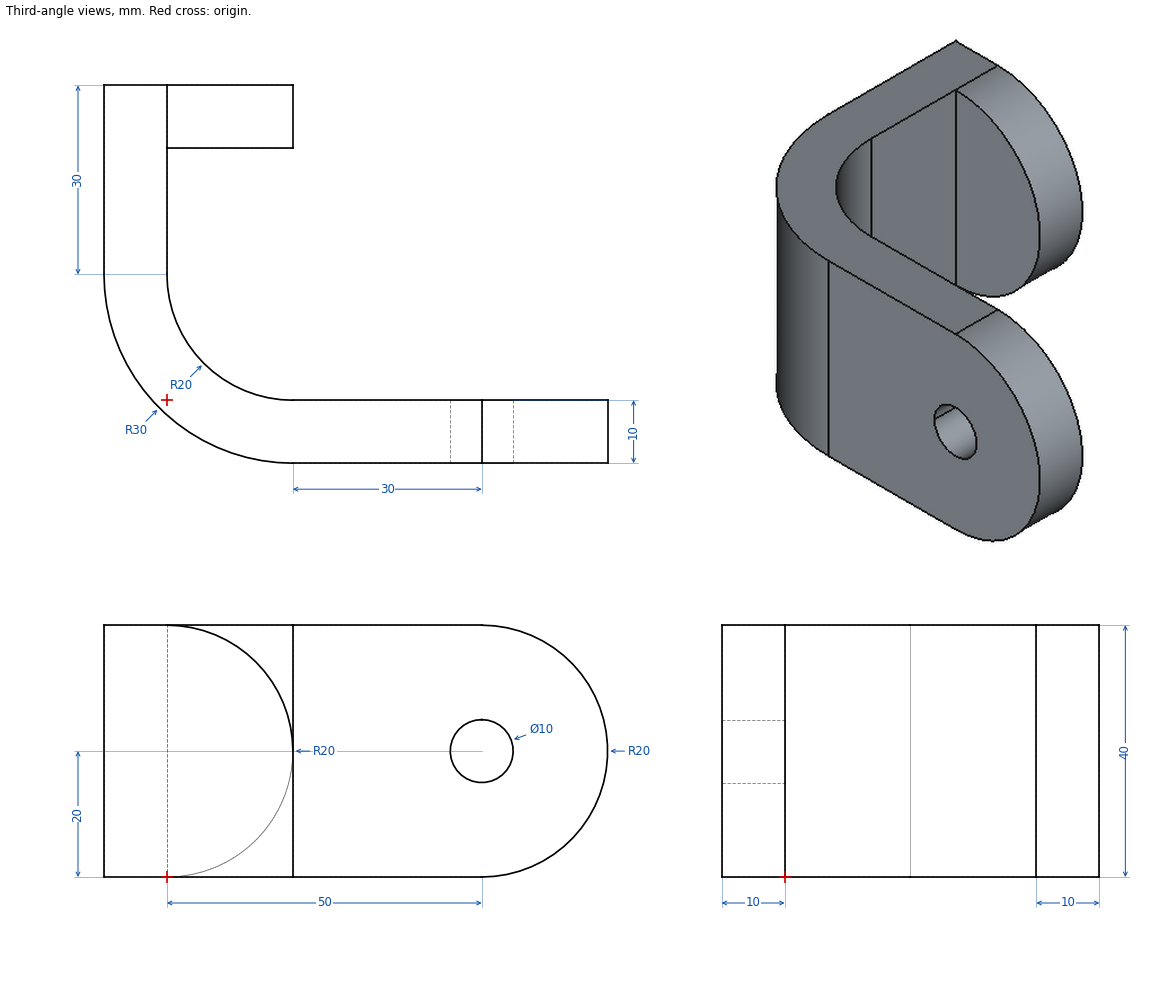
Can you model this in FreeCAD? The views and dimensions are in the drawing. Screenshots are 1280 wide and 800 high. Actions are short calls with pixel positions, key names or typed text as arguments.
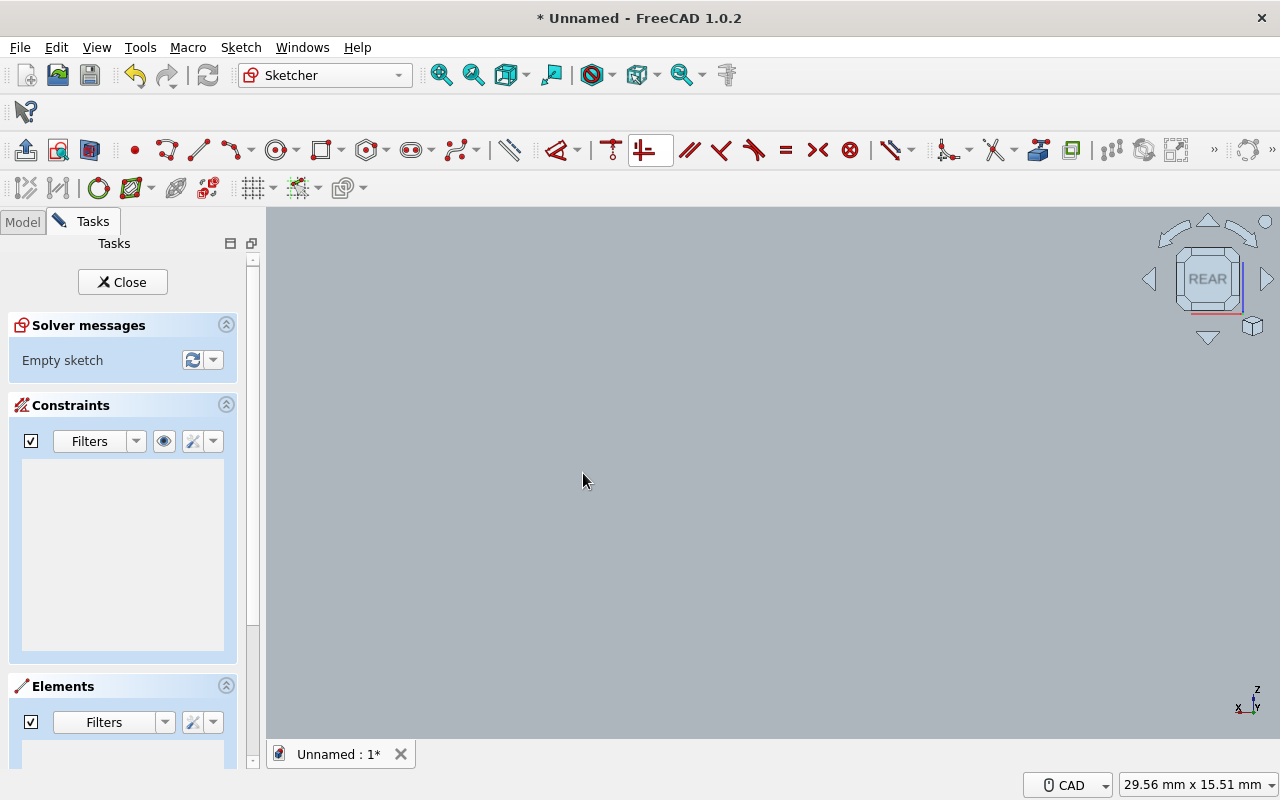
key(g)
key(c)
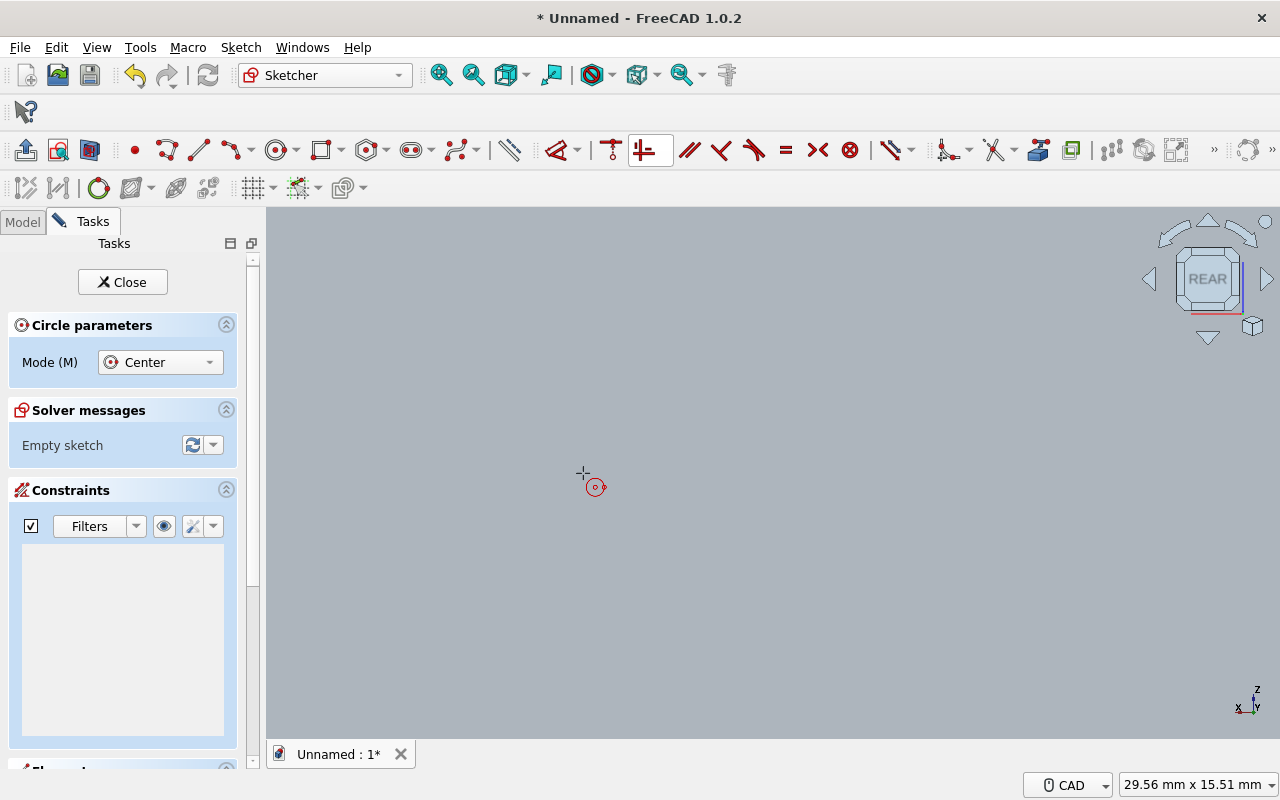
click(702, 470)
click(823, 349)
key(Escape)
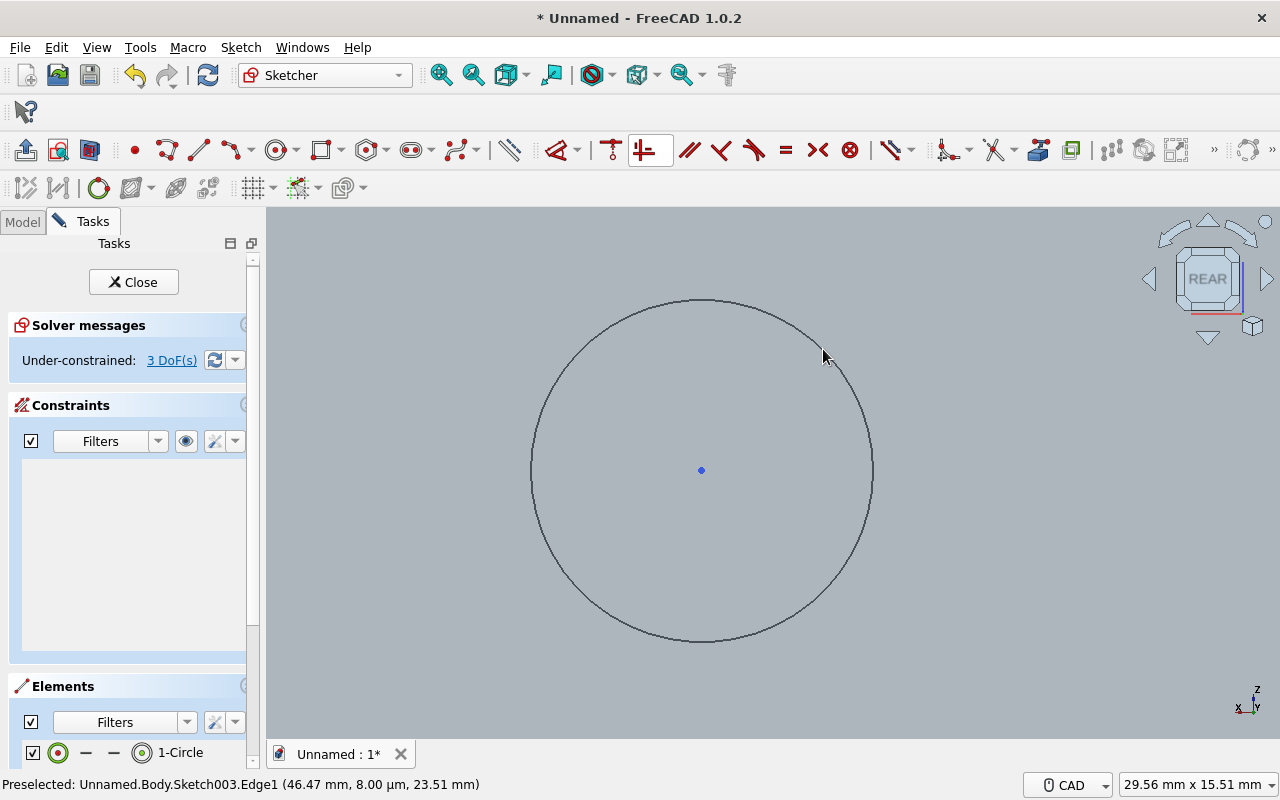
click(556, 150)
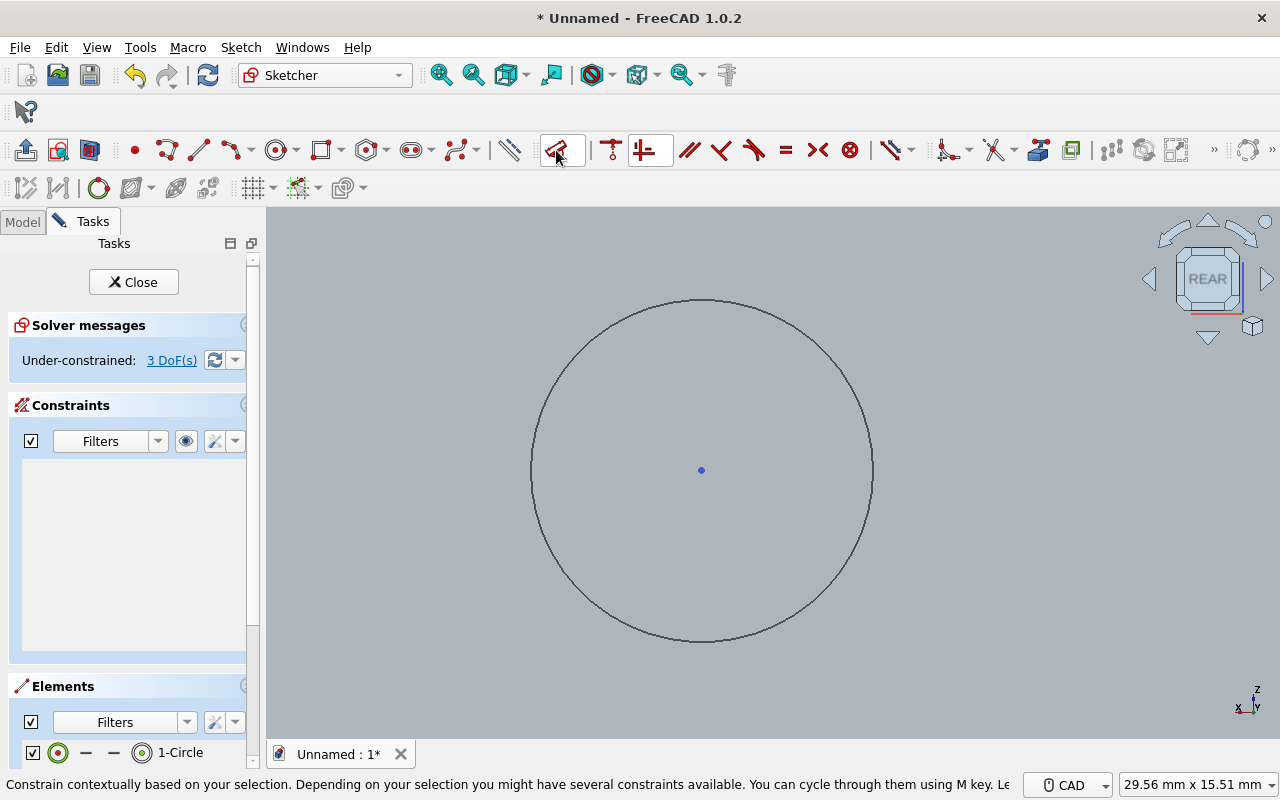
click(823, 350)
click(846, 327)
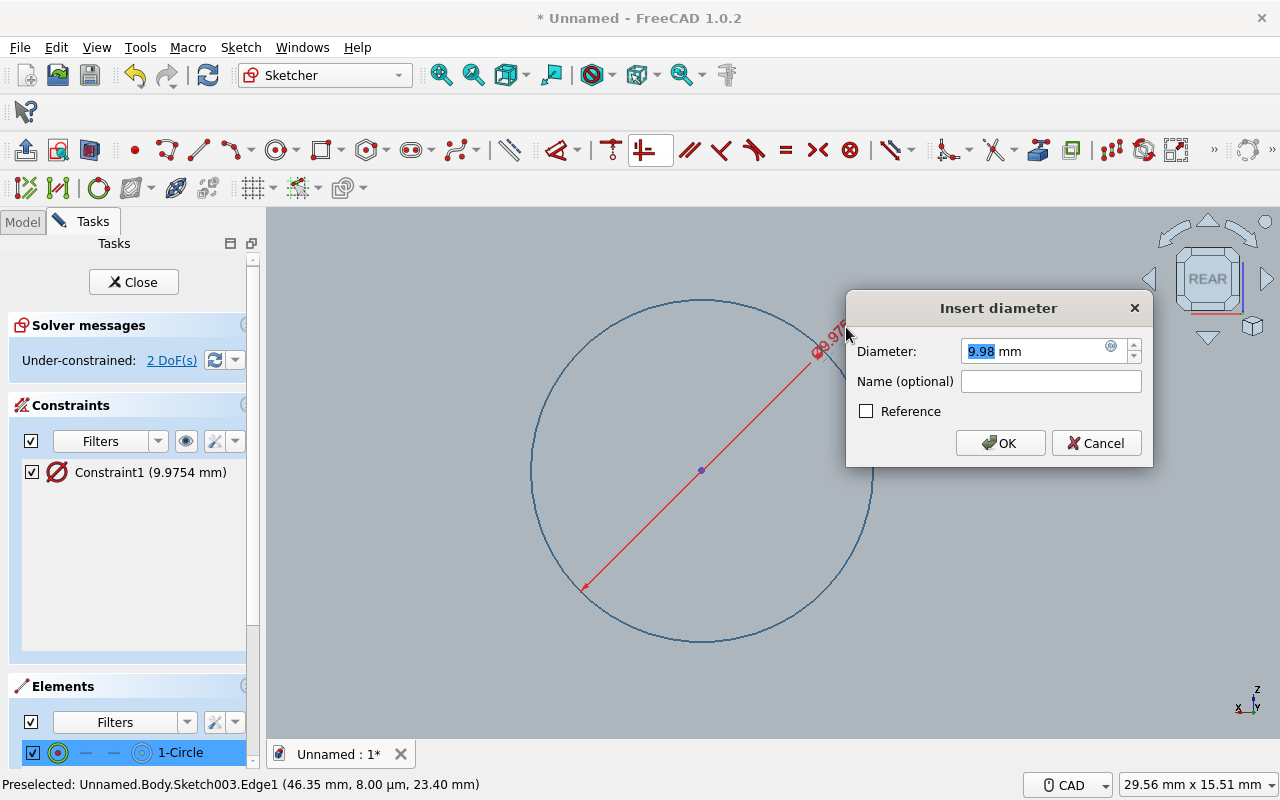
text(10)
key(Return)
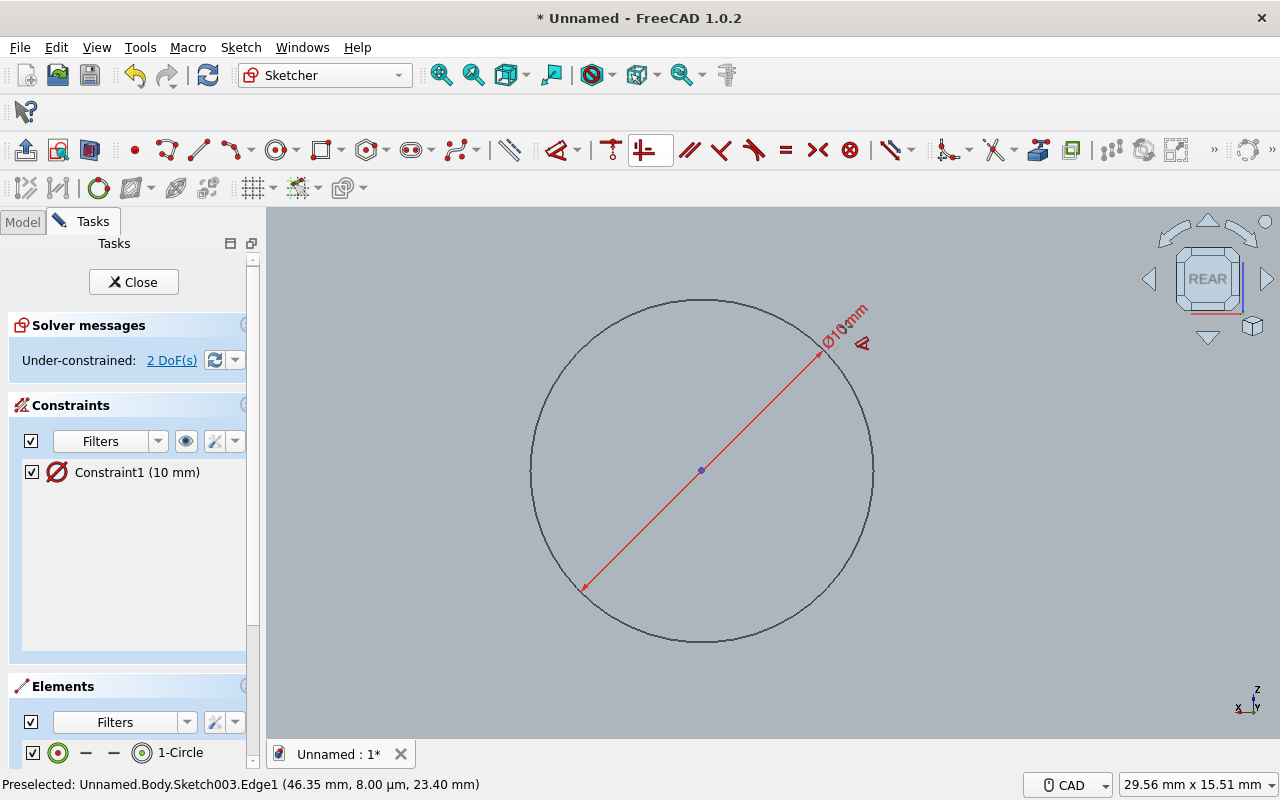
click(702, 471)
click(908, 437)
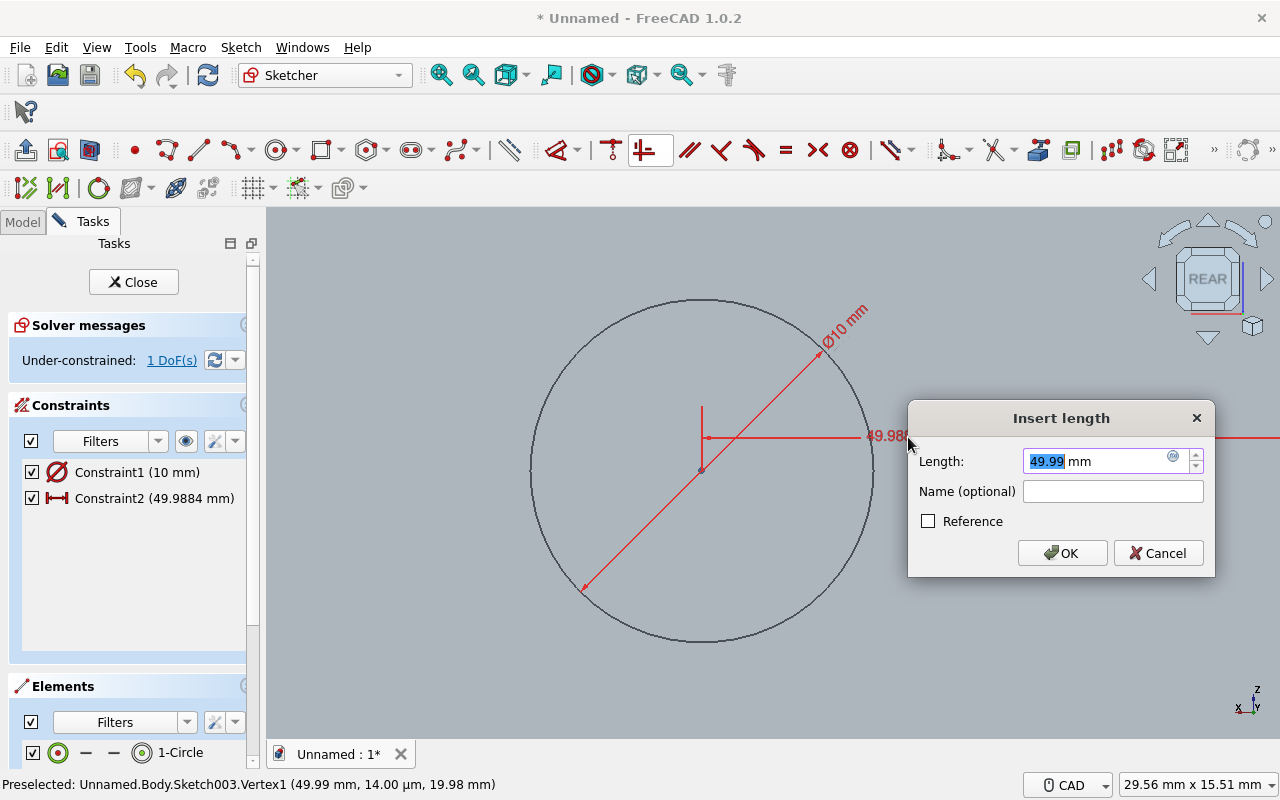
text(50)
key(Return)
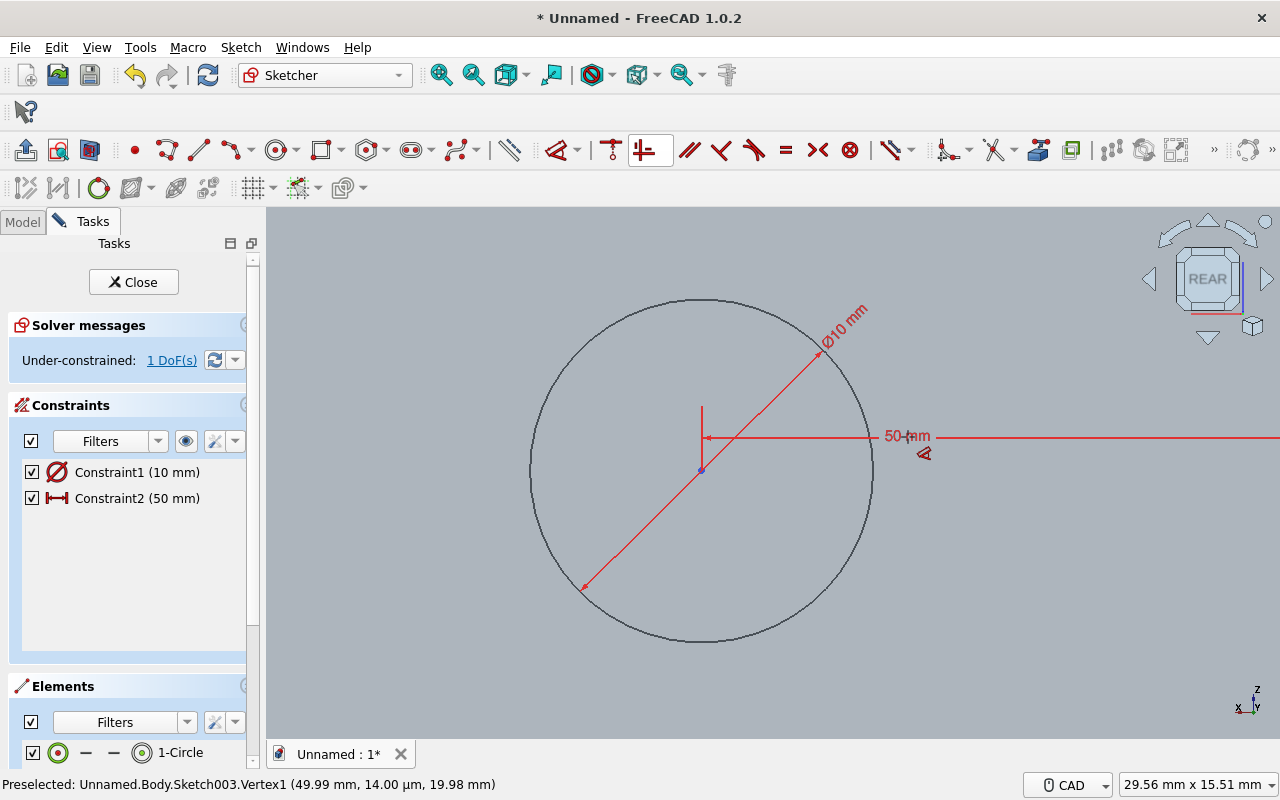
click(702, 471)
click(668, 591)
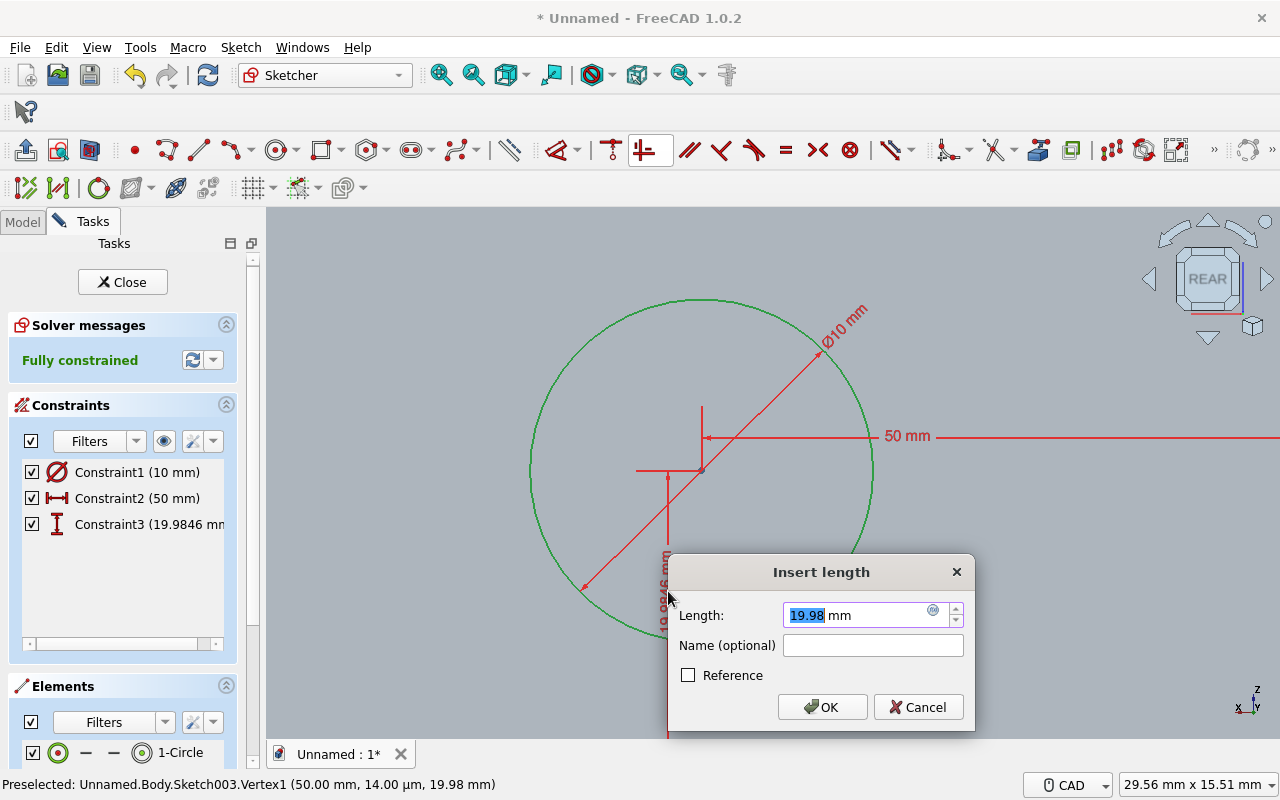
text(20)
key(Return)
key(Escape)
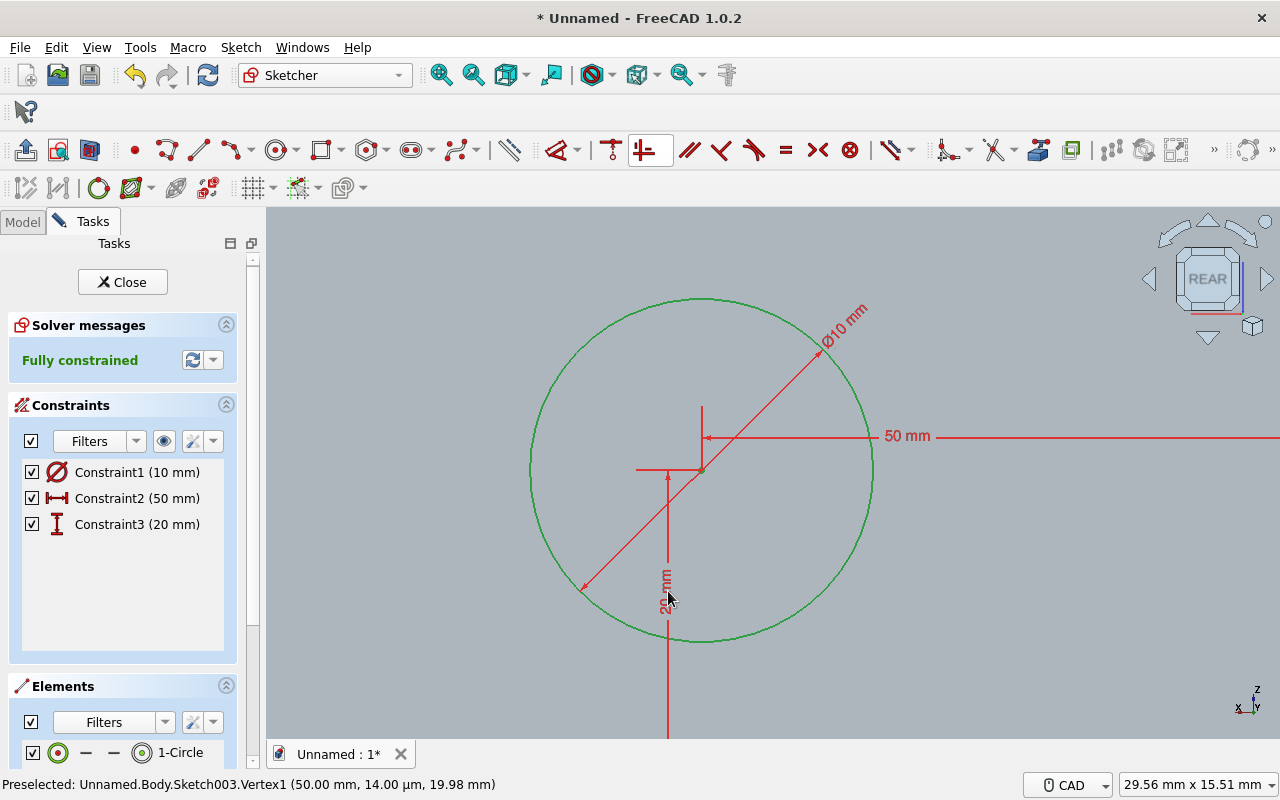
click(123, 282)